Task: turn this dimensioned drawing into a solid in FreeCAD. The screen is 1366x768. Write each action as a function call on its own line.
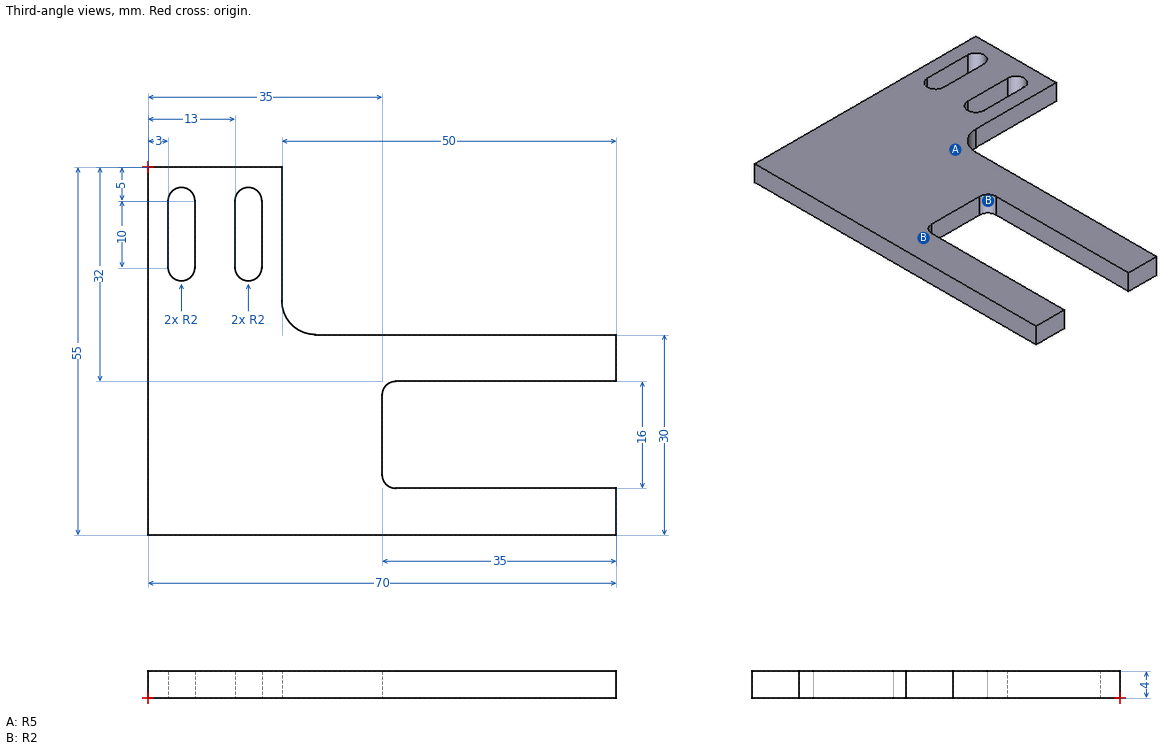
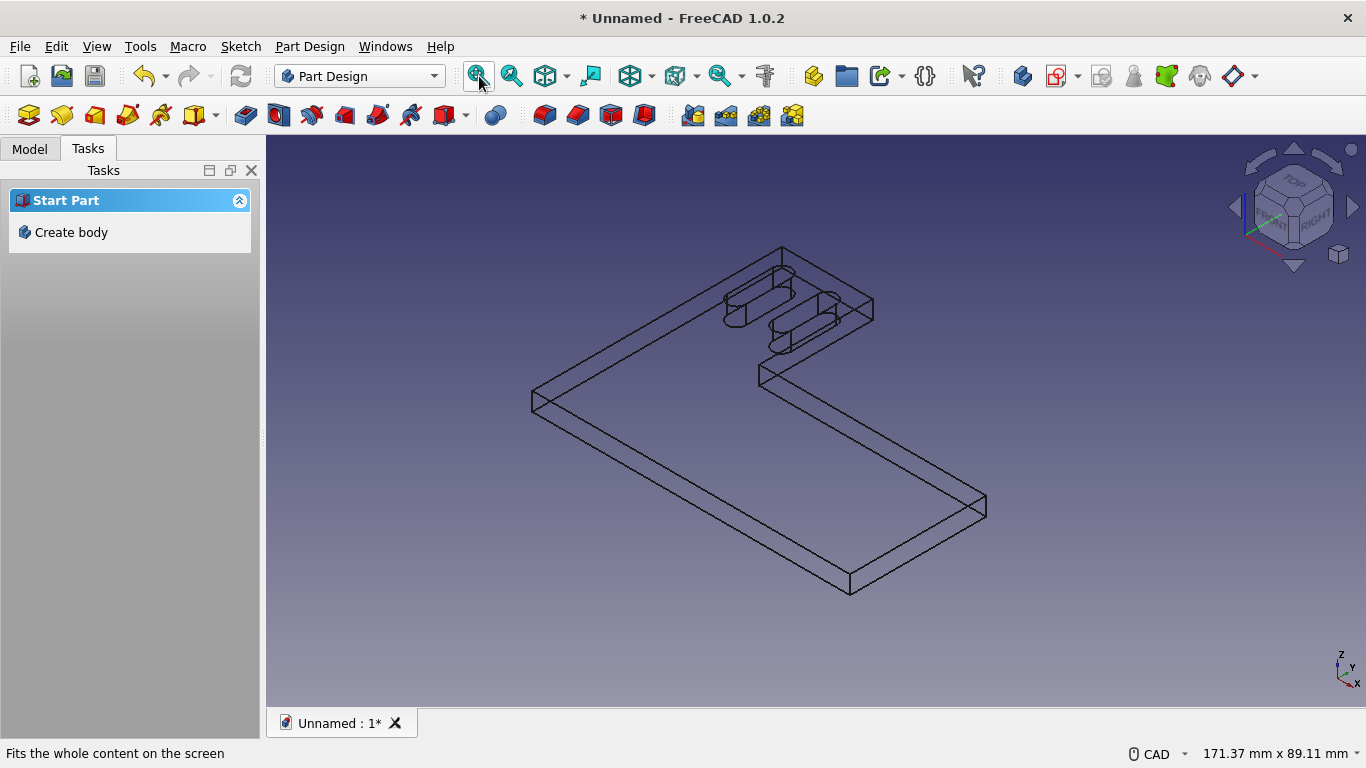
click(759, 374)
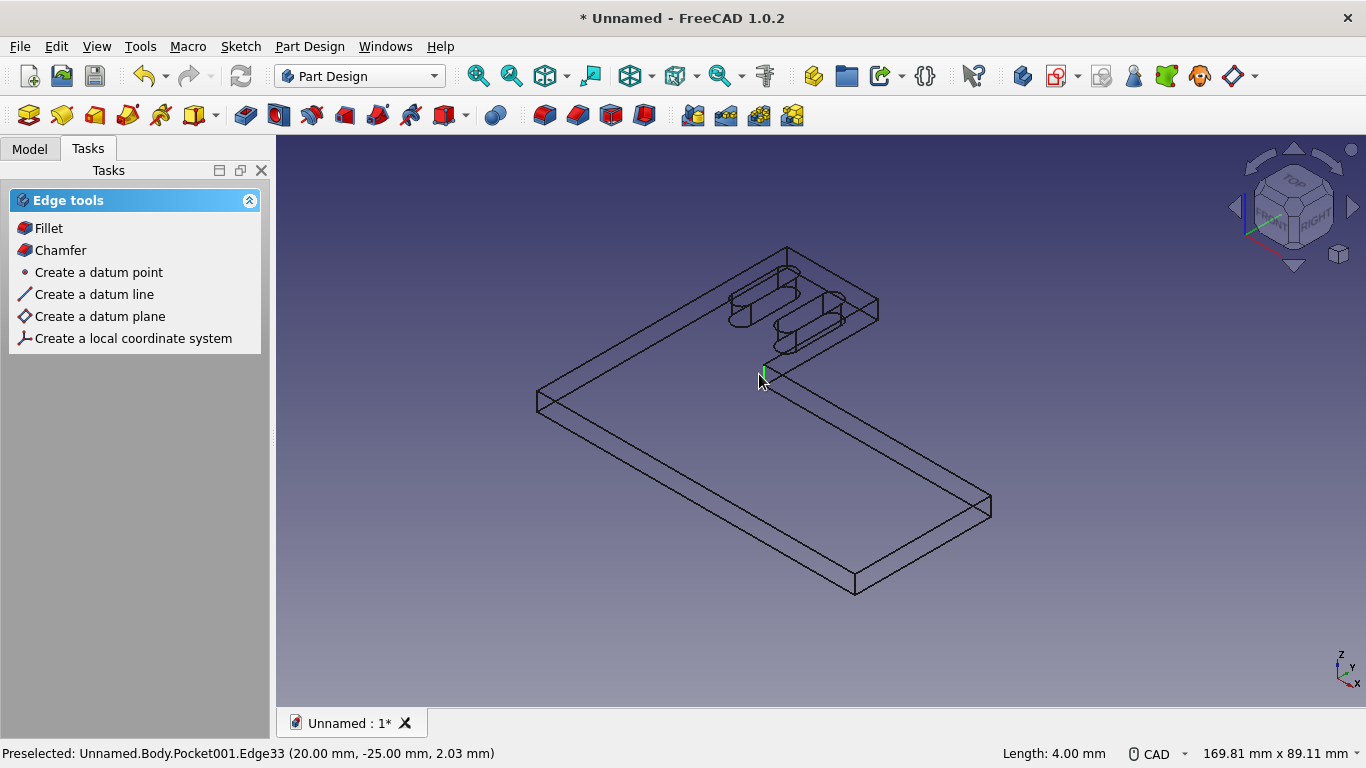
key(v)
key(1)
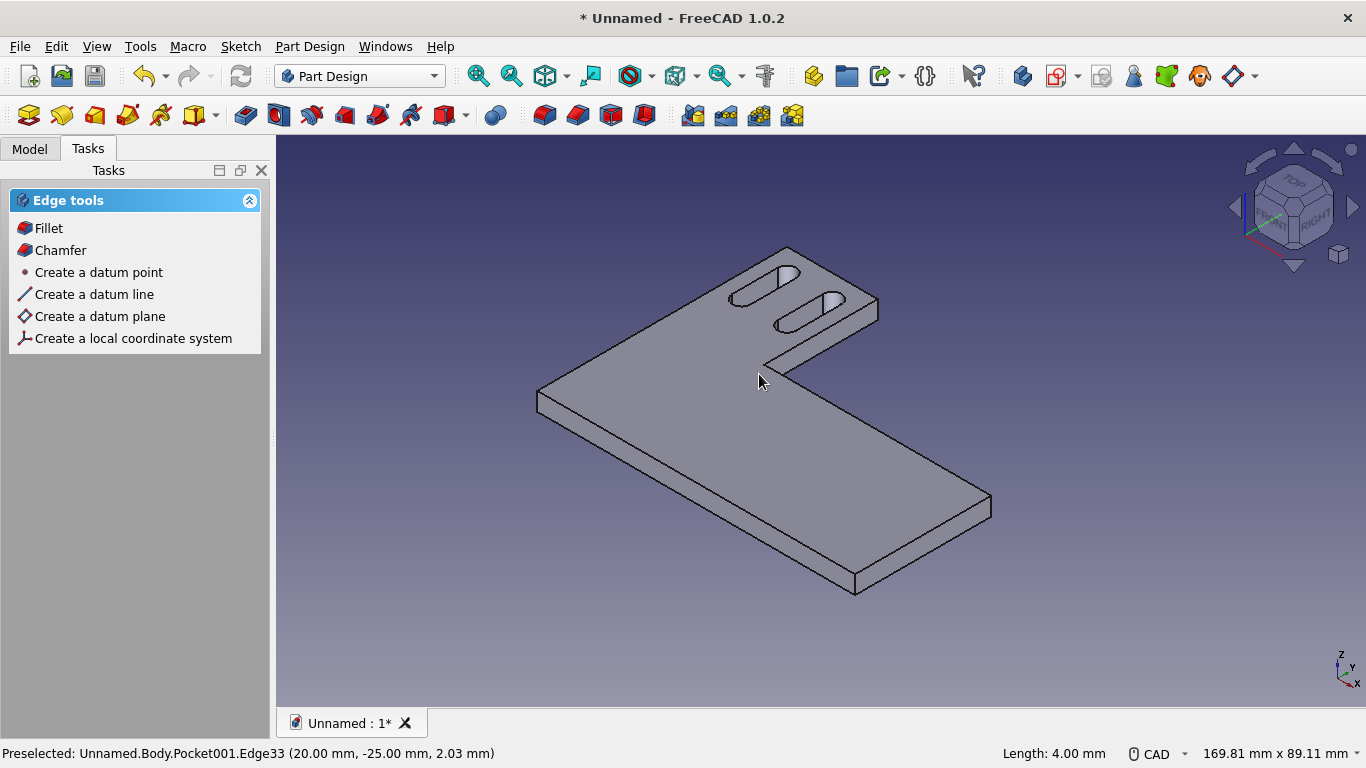
click(545, 116)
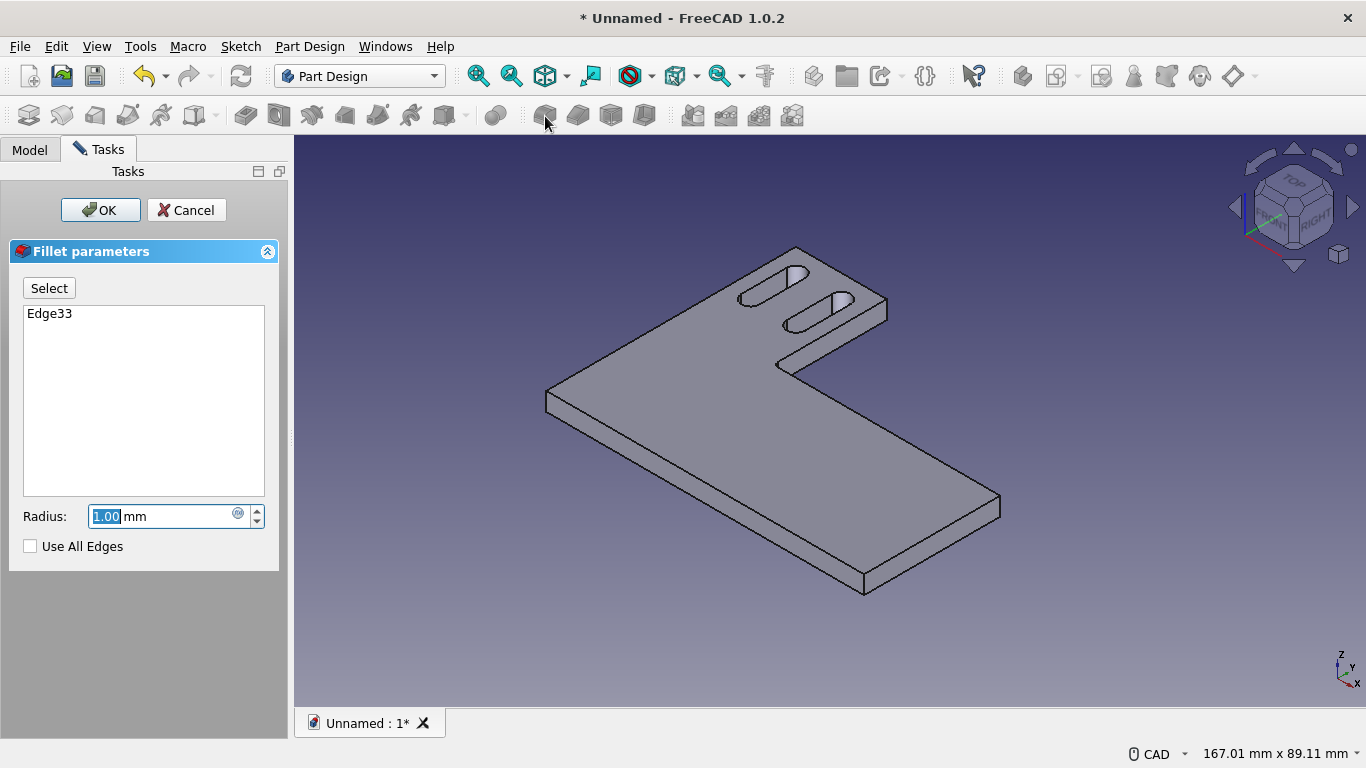
text(5)
key(Tab)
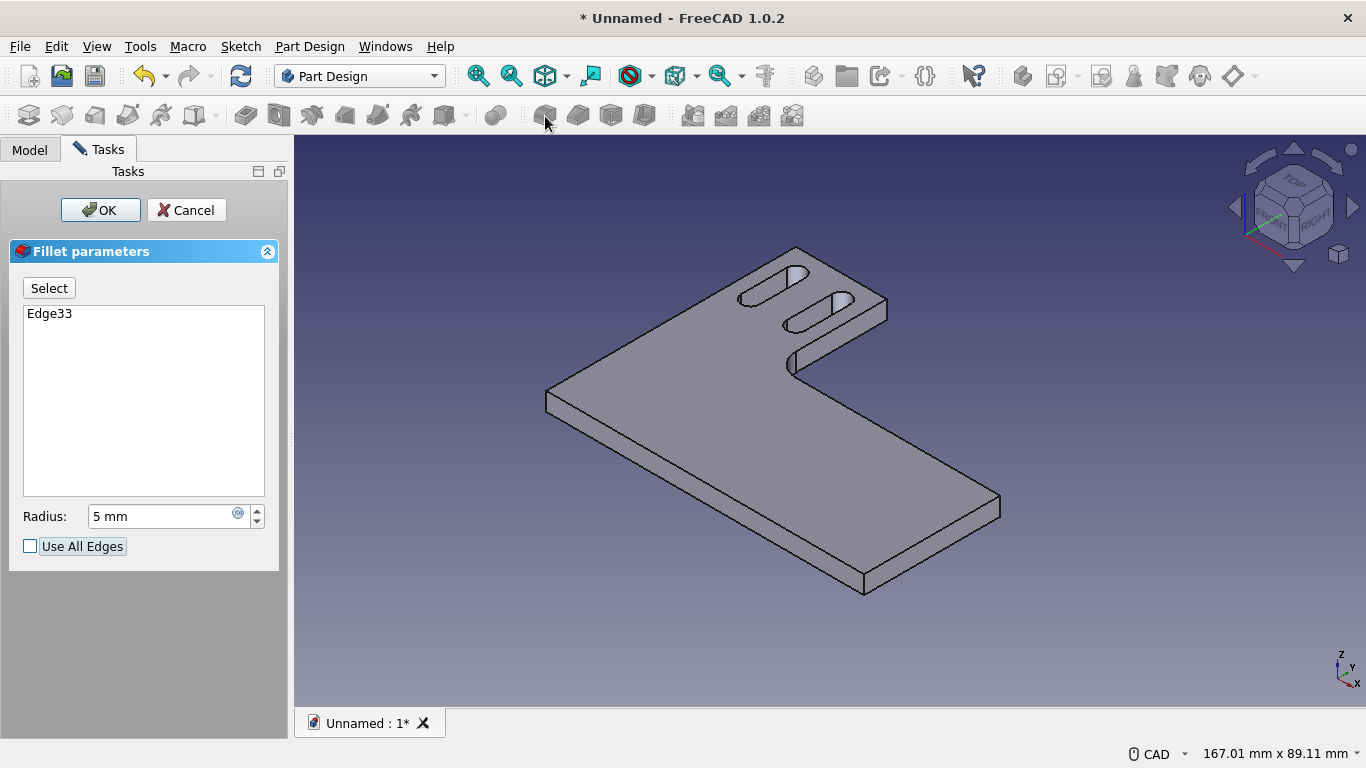
click(101, 210)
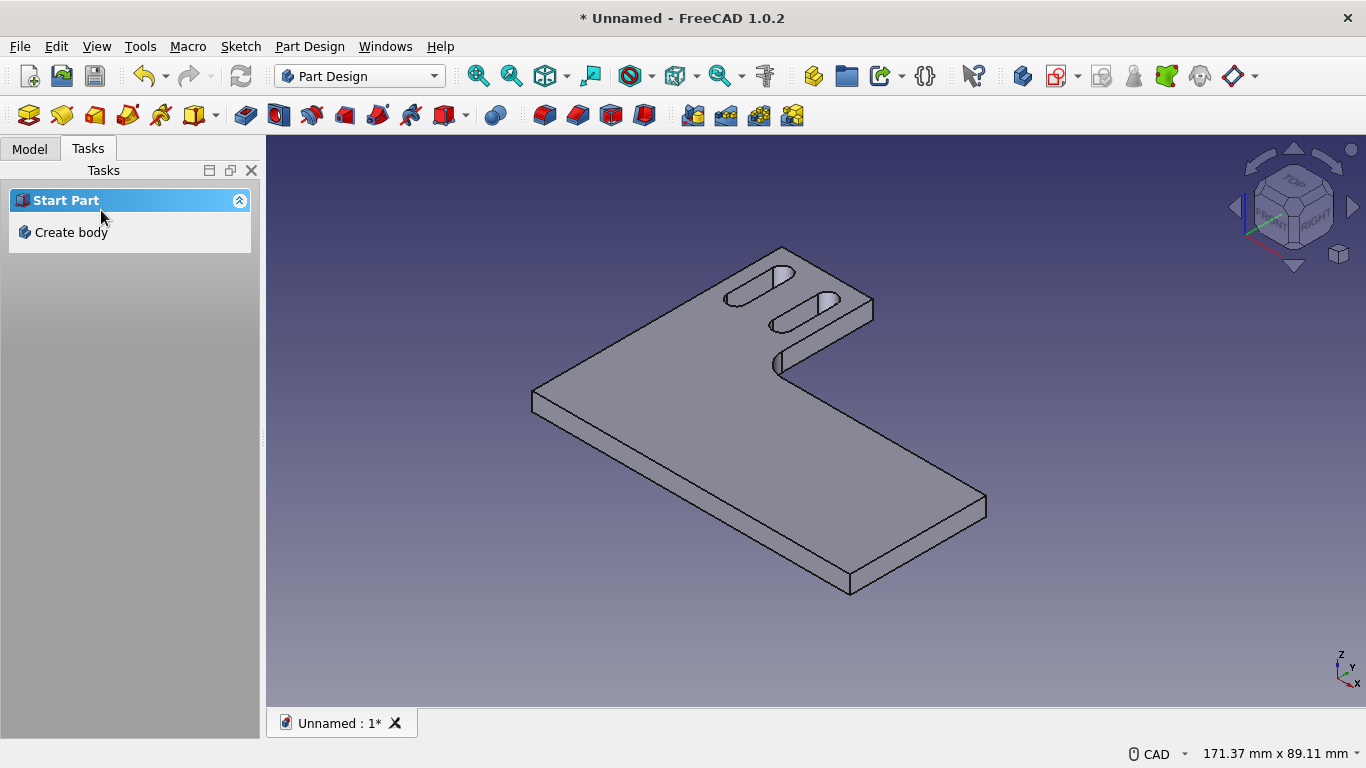
click(690, 378)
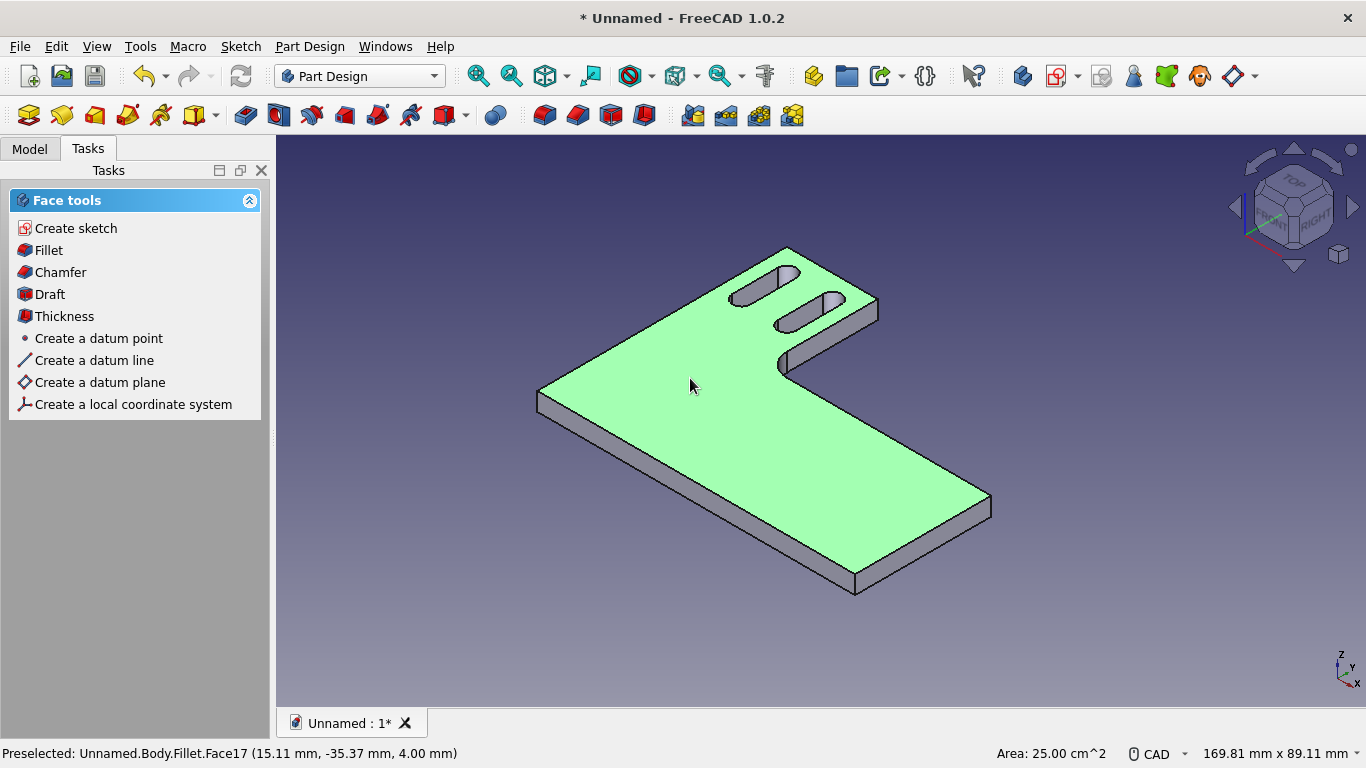
click(1056, 76)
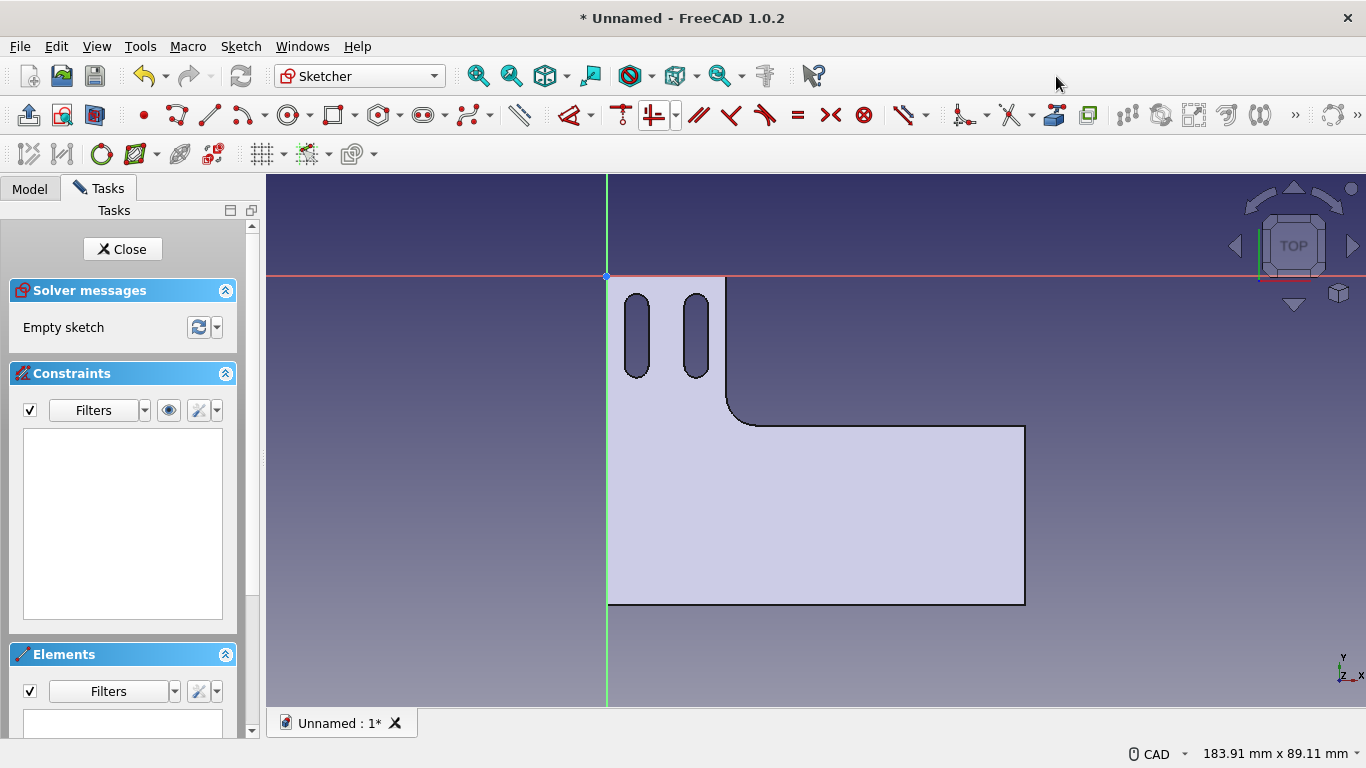
click(332, 116)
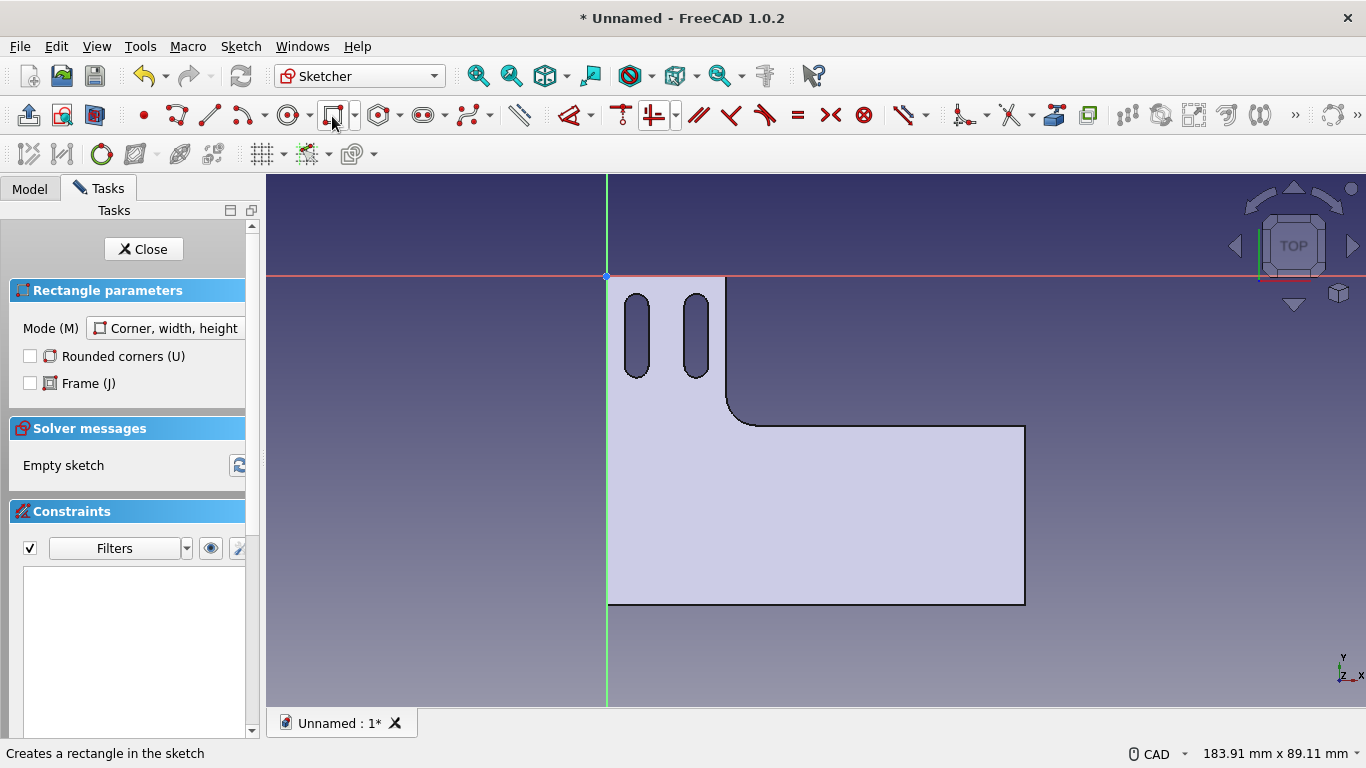
click(816, 467)
move(1025, 563)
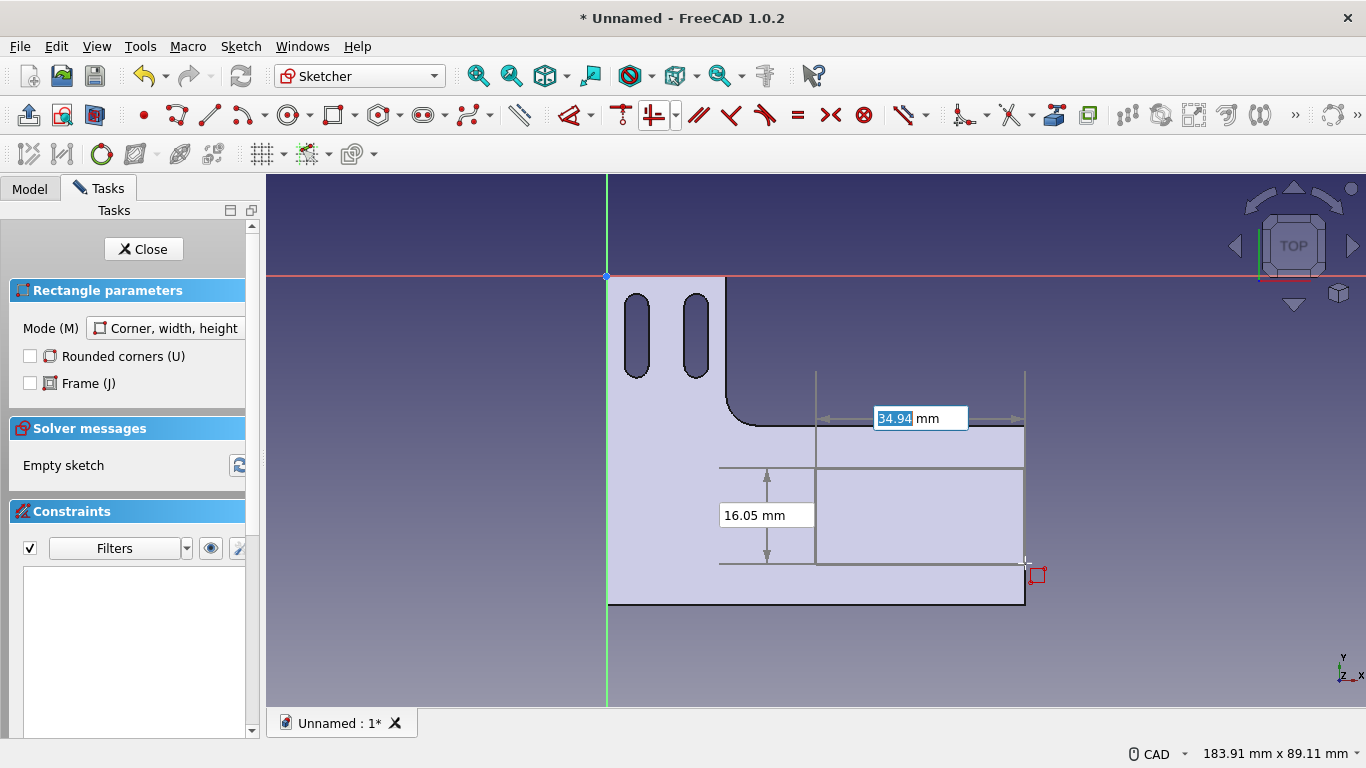
text(35)
key(Tab)
text(16)
key(Return)
key(Escape)